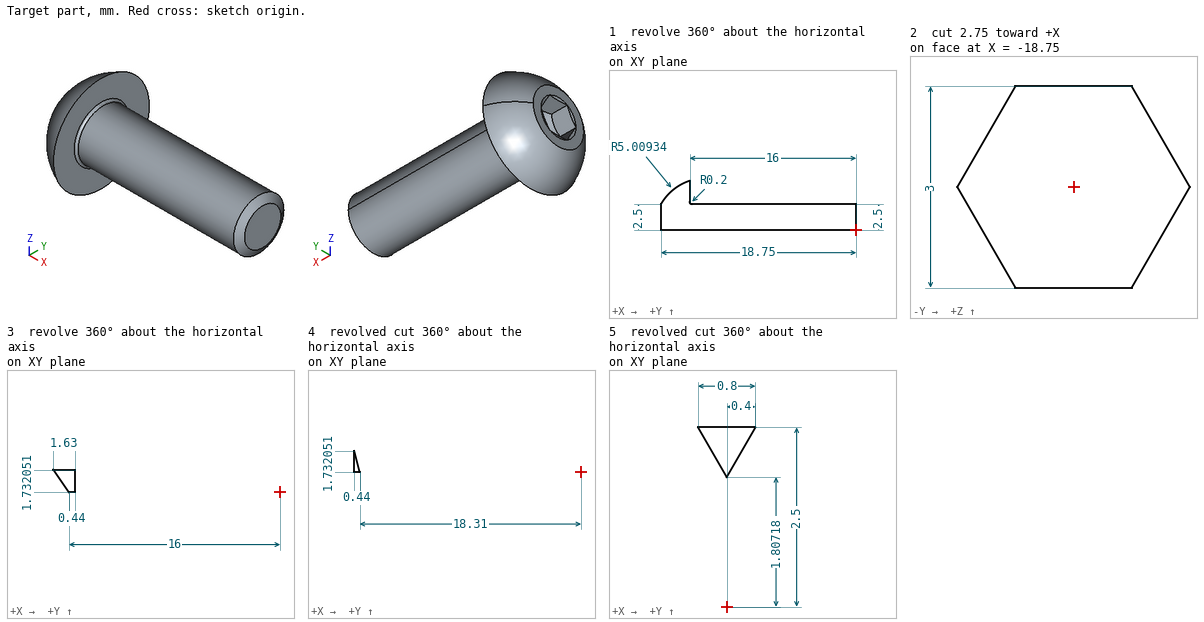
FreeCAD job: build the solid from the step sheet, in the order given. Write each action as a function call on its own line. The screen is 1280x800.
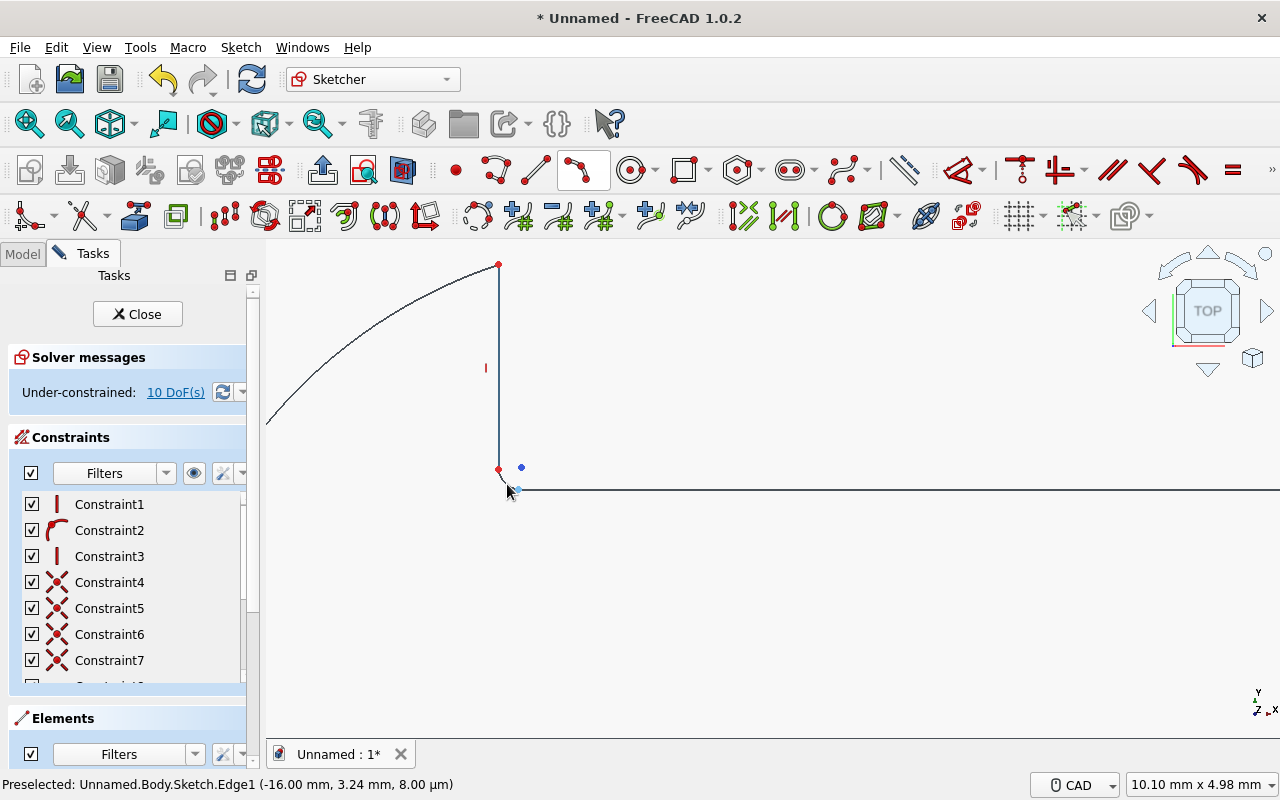
click(505, 483)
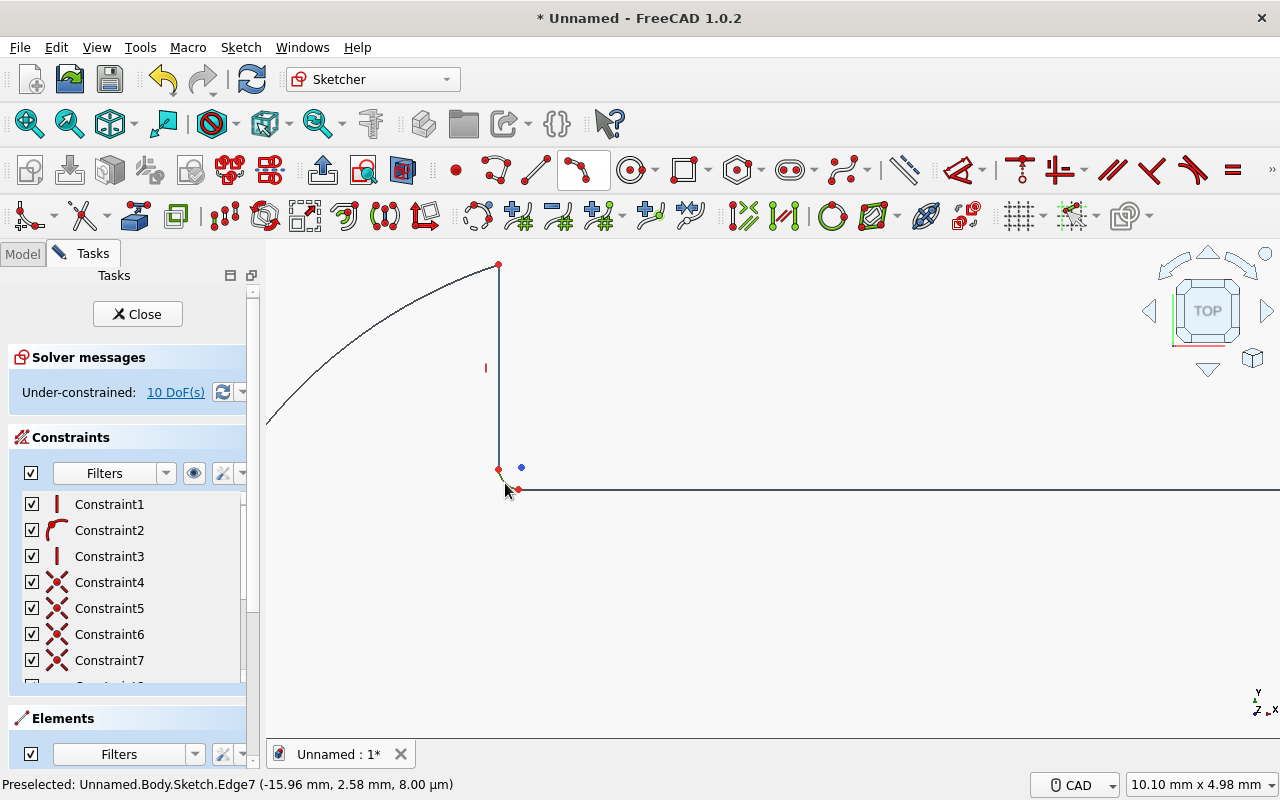
click(1194, 170)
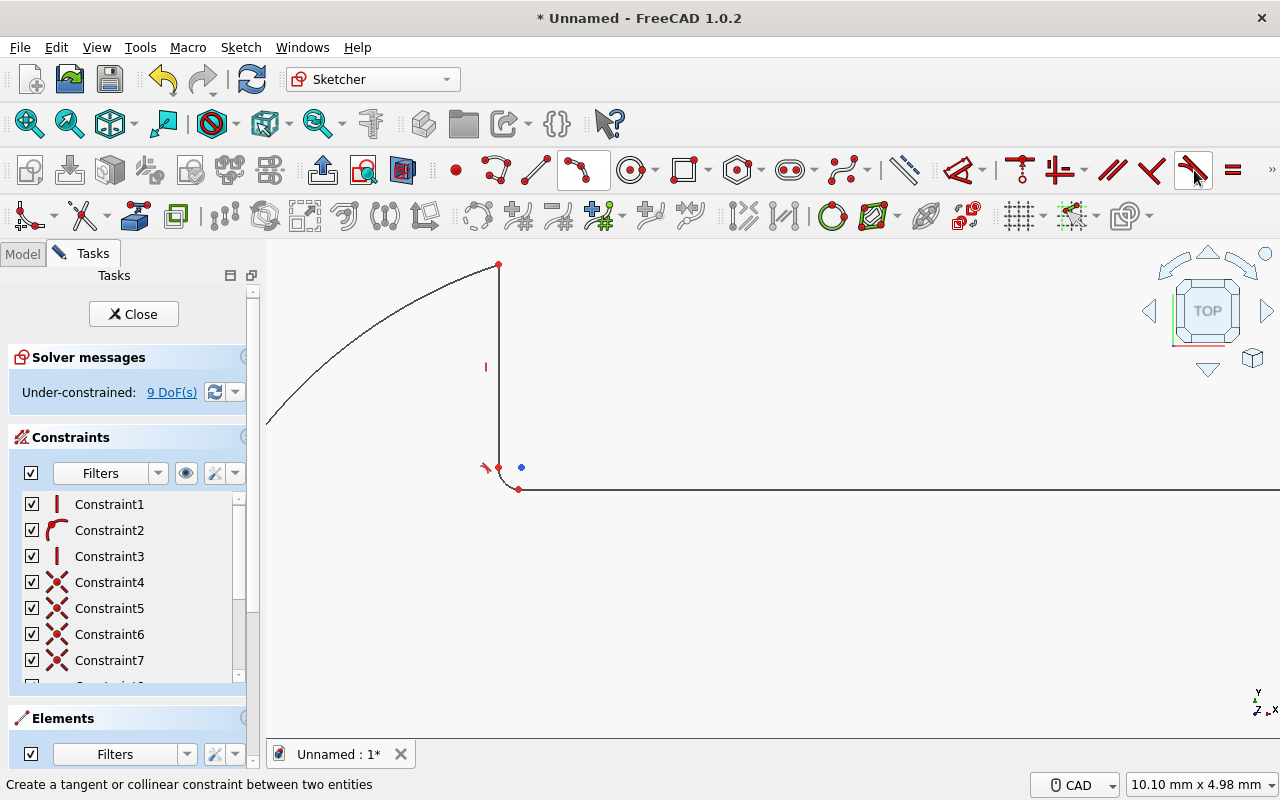
click(986, 490)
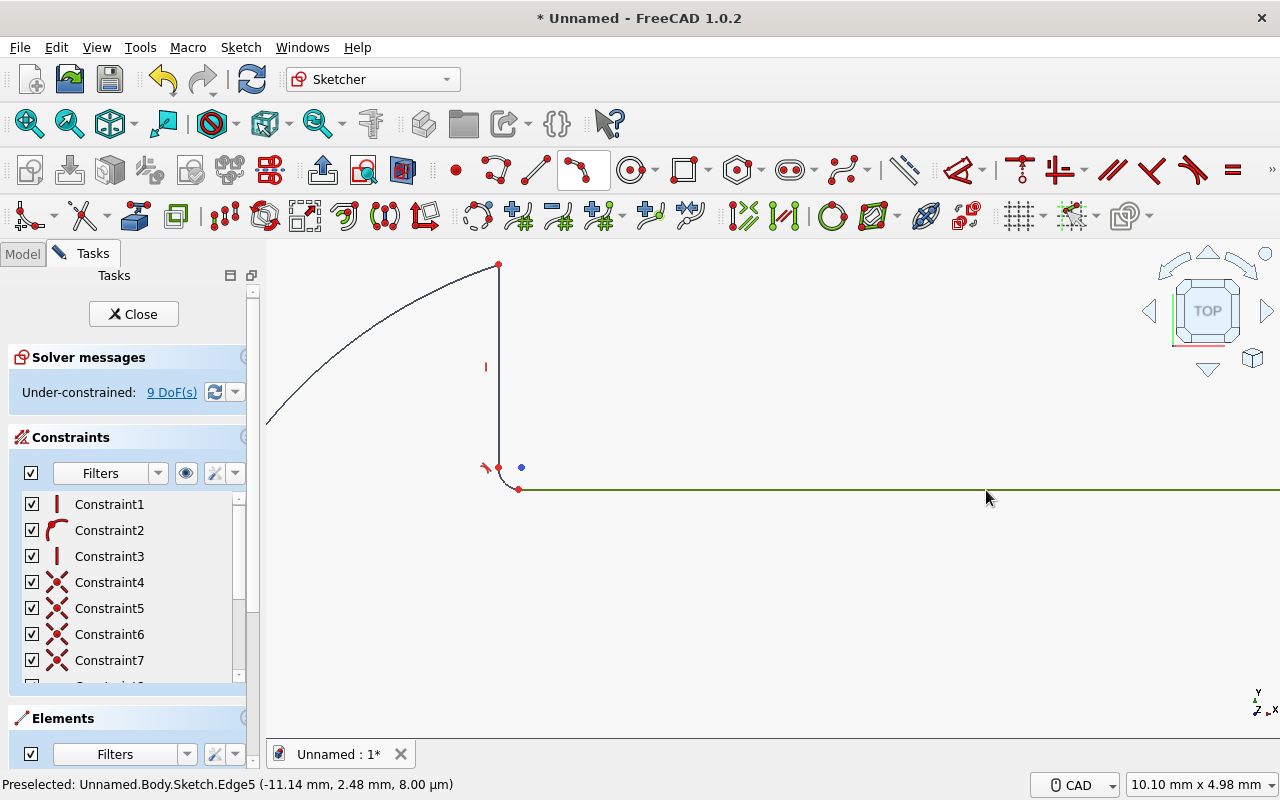
scroll(501, 477, up, 2)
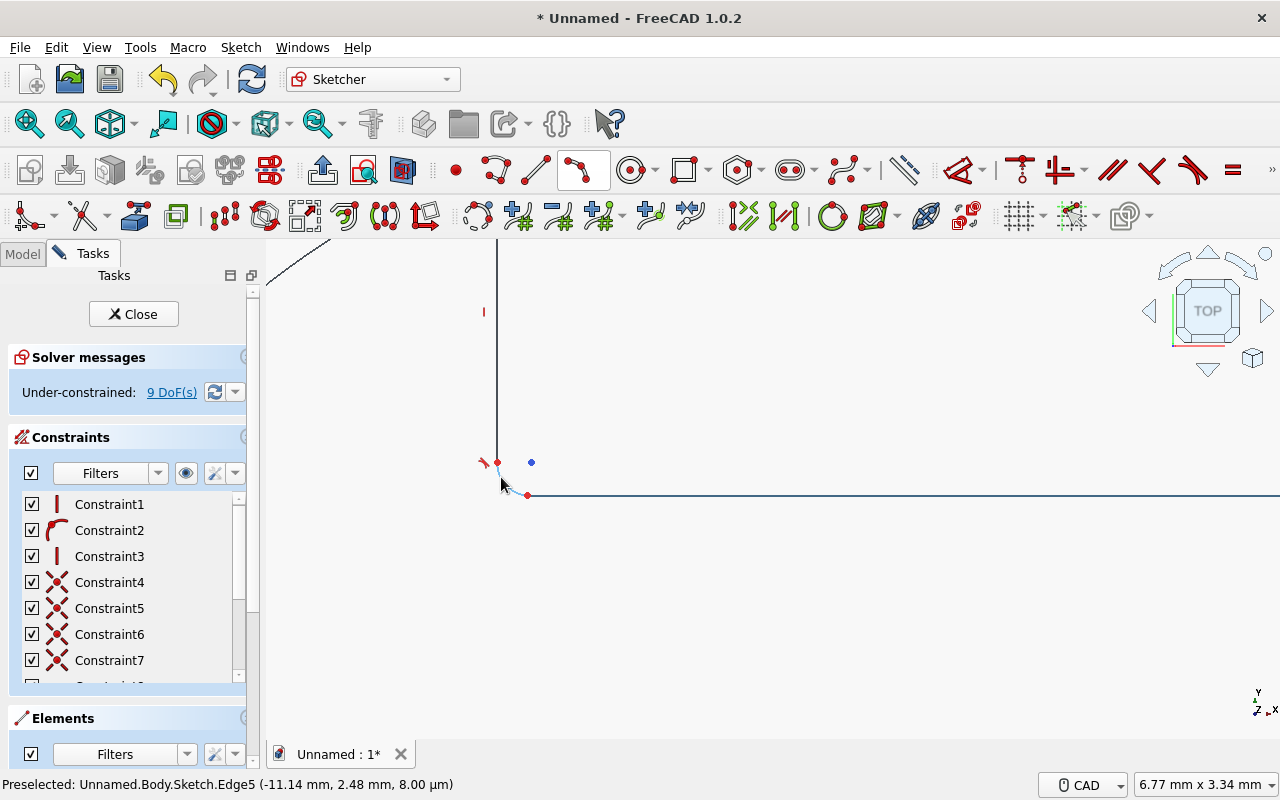
click(500, 477)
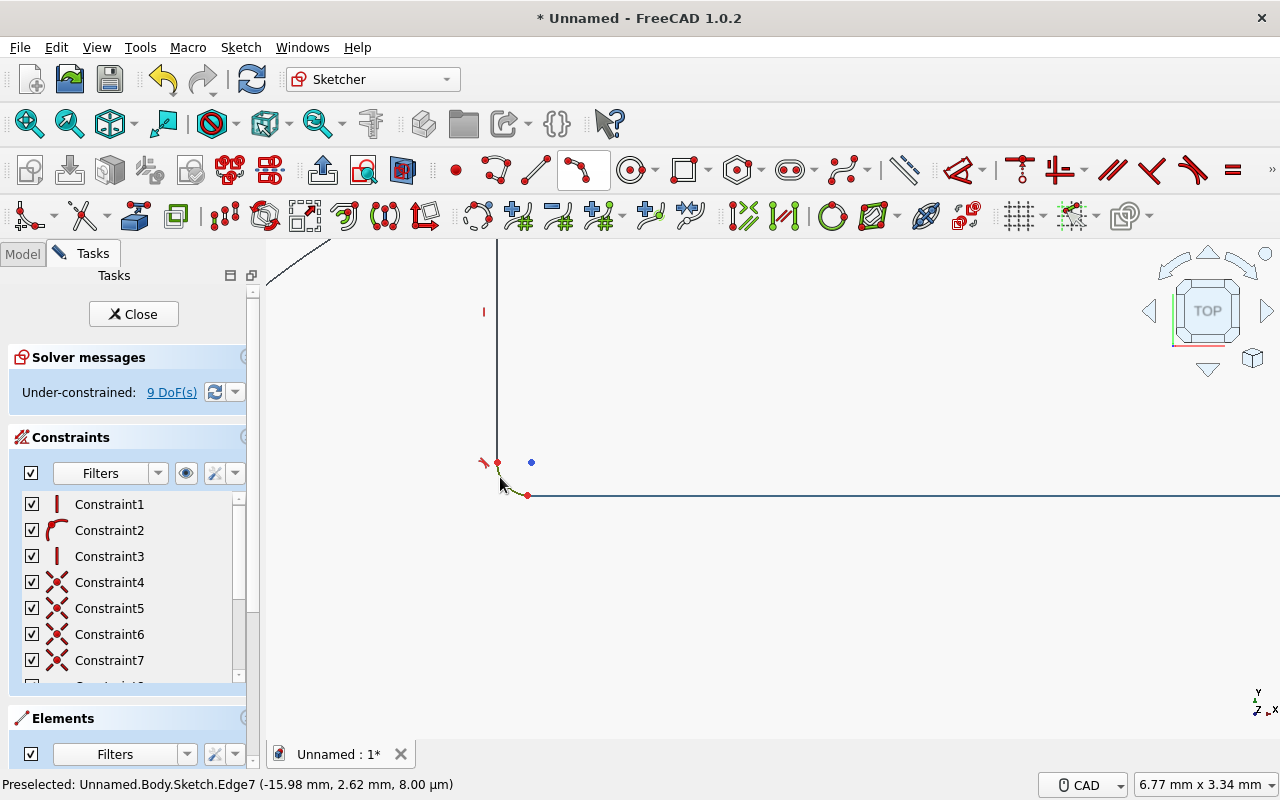
click(1194, 170)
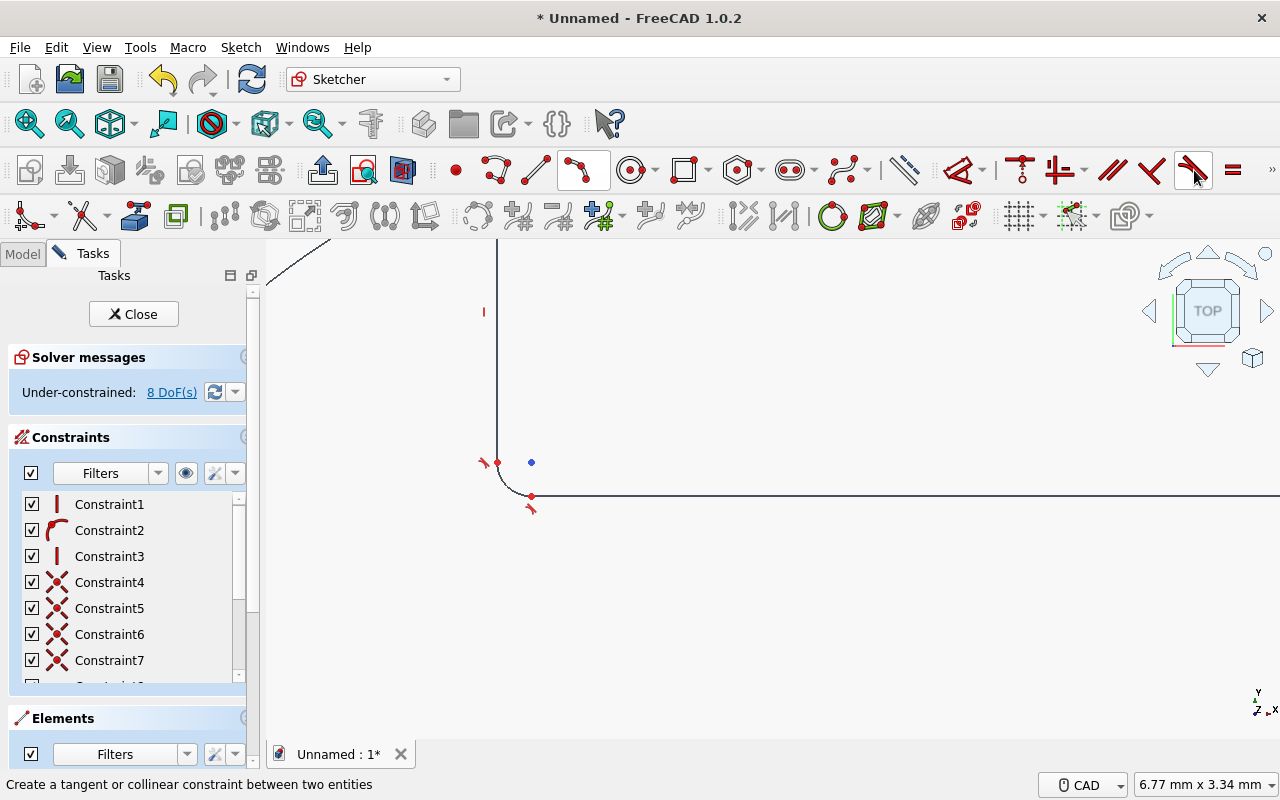
scroll(506, 483, down, 8)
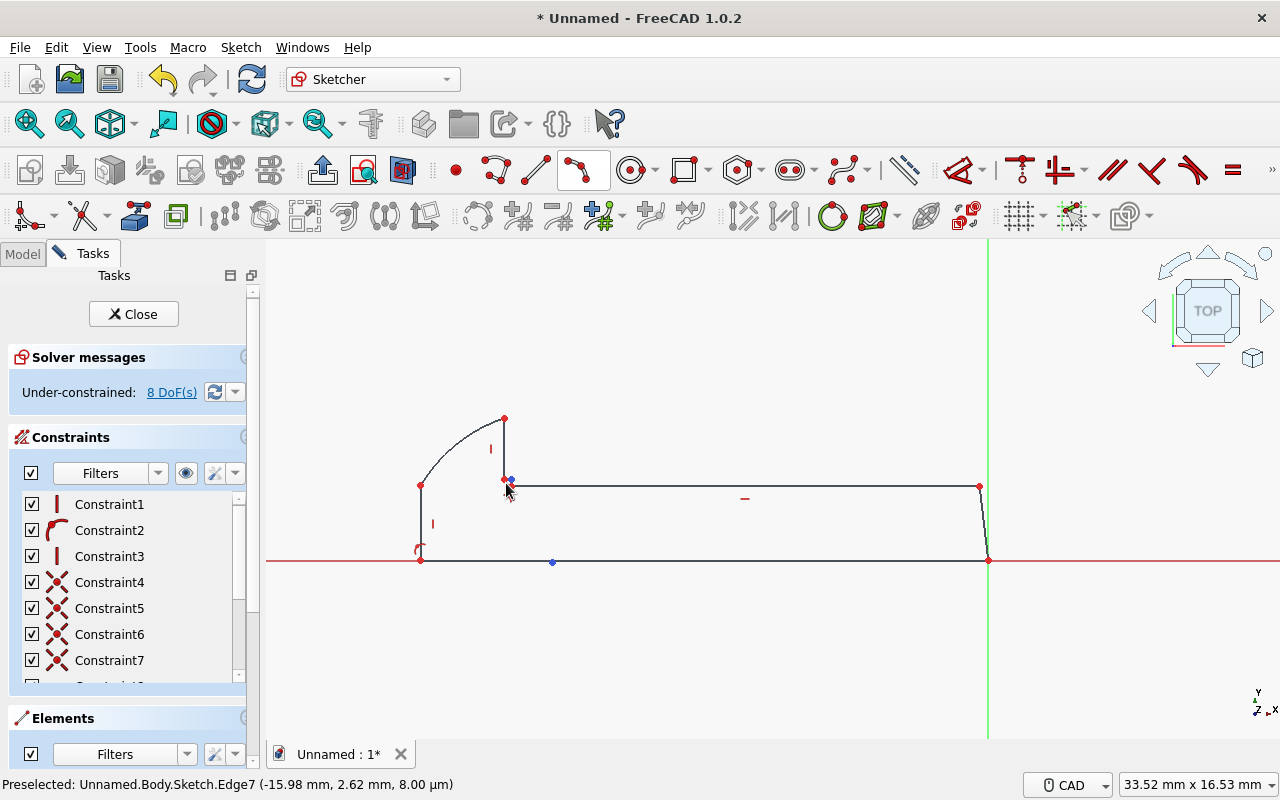
scroll(986, 538, up, 9)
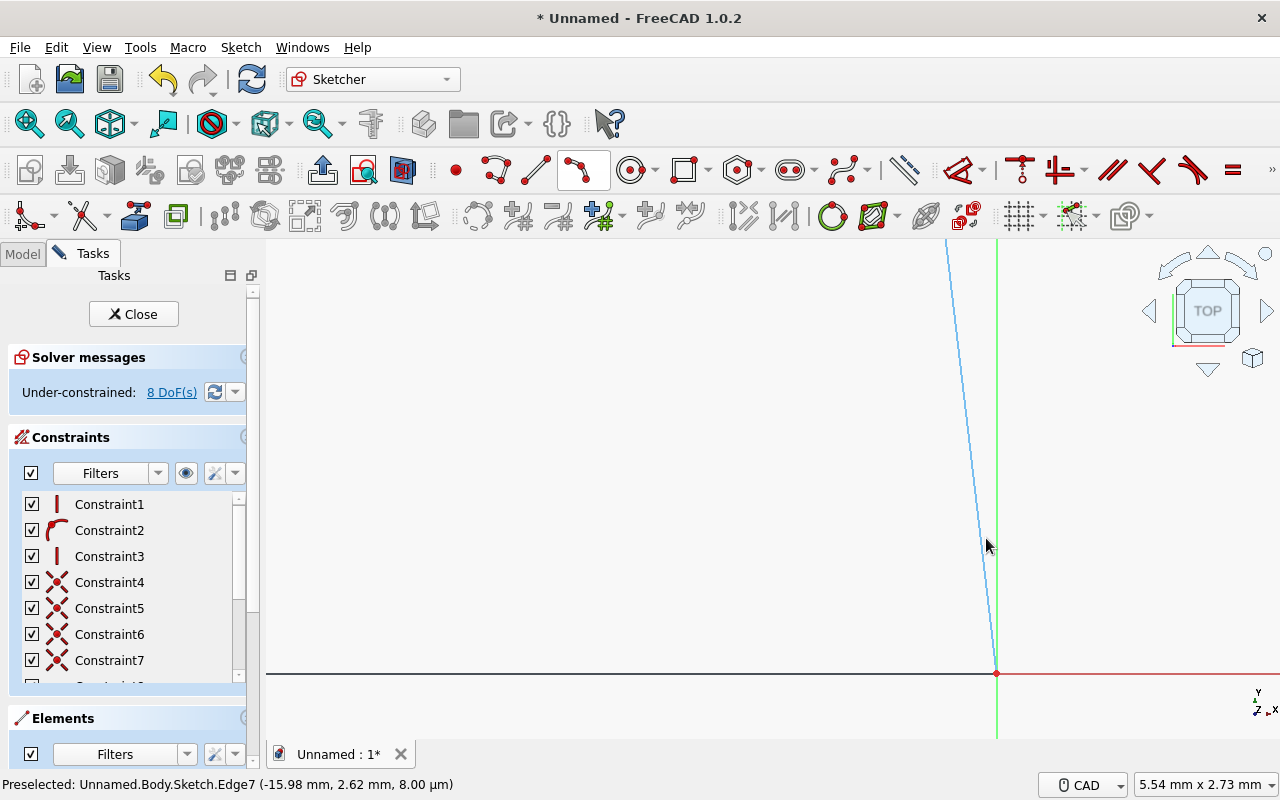
click(981, 538)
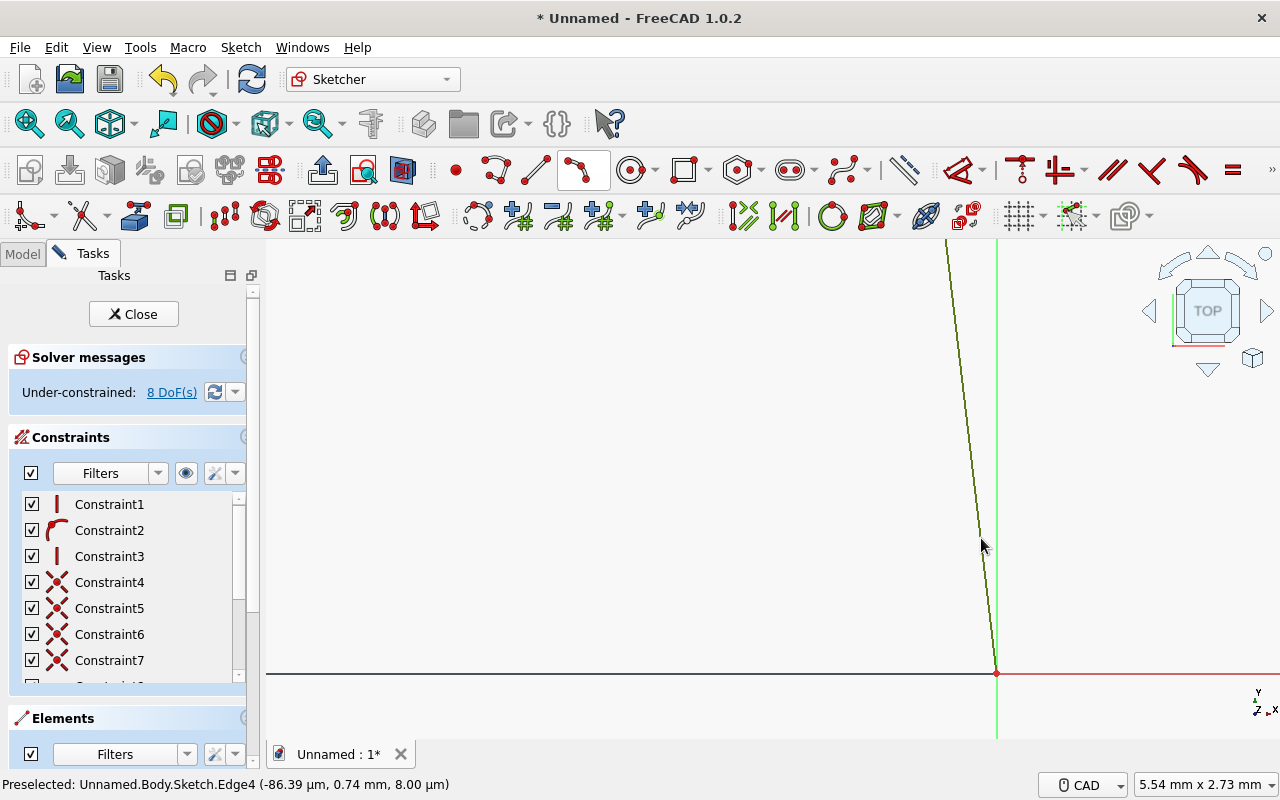
click(1086, 170)